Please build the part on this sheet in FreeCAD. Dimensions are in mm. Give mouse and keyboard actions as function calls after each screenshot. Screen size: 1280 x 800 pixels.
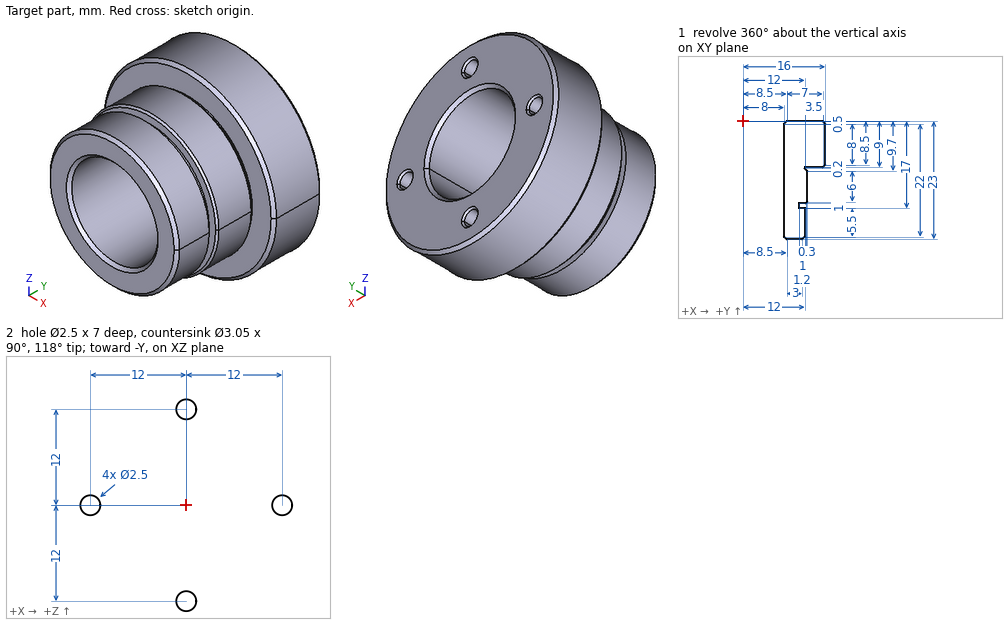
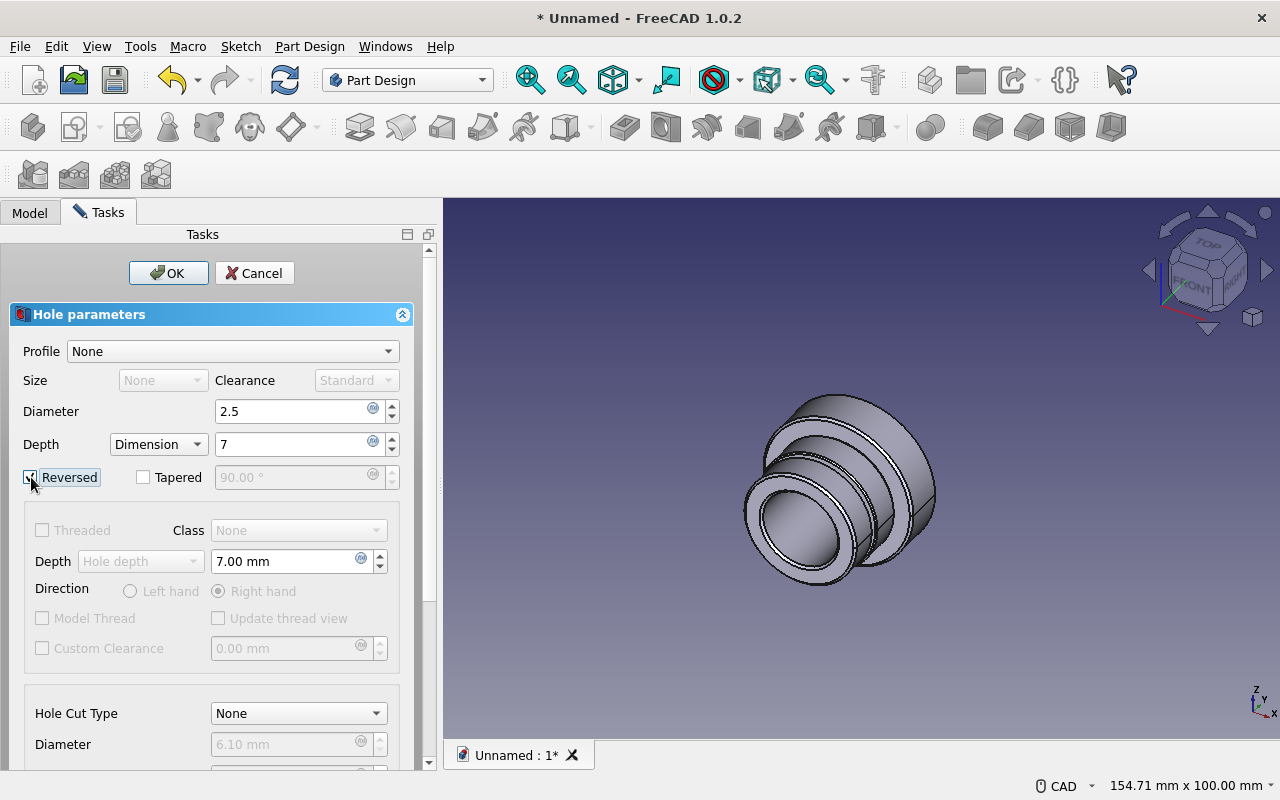
click(300, 714)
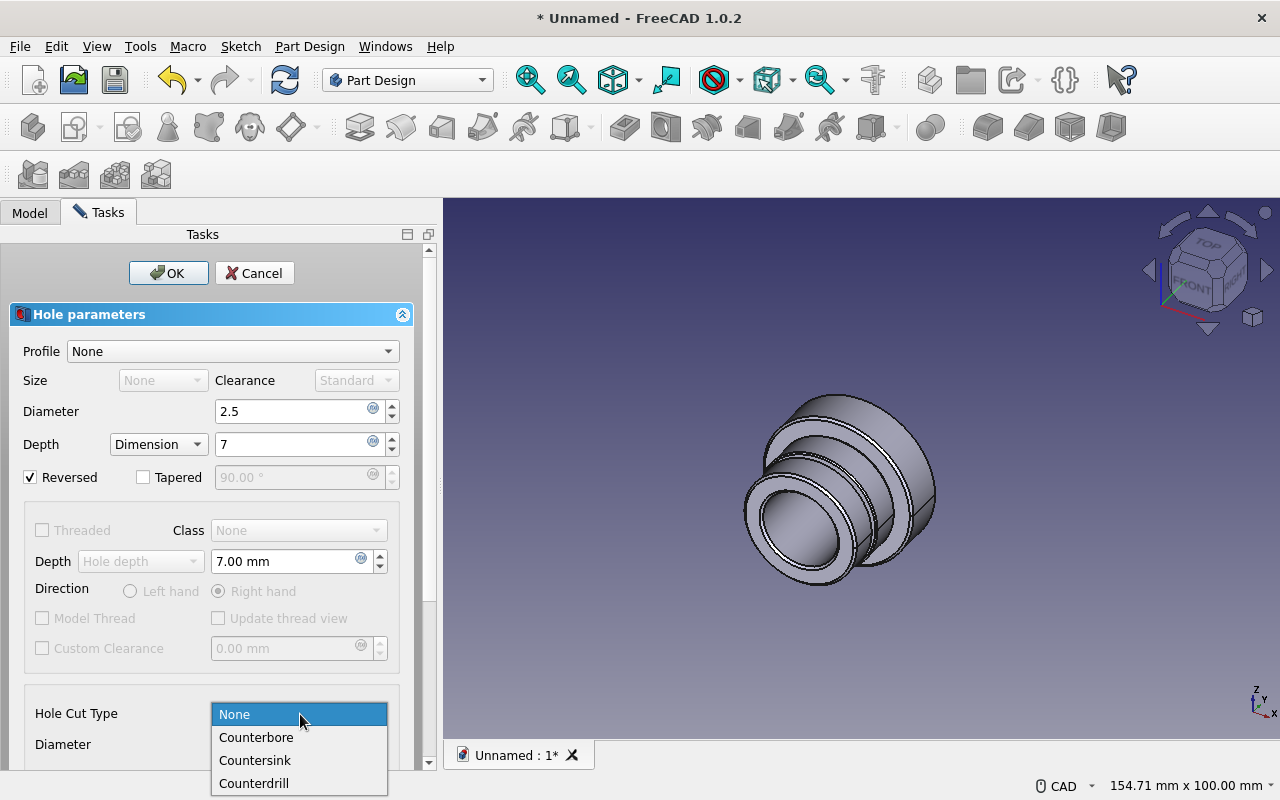
click(298, 760)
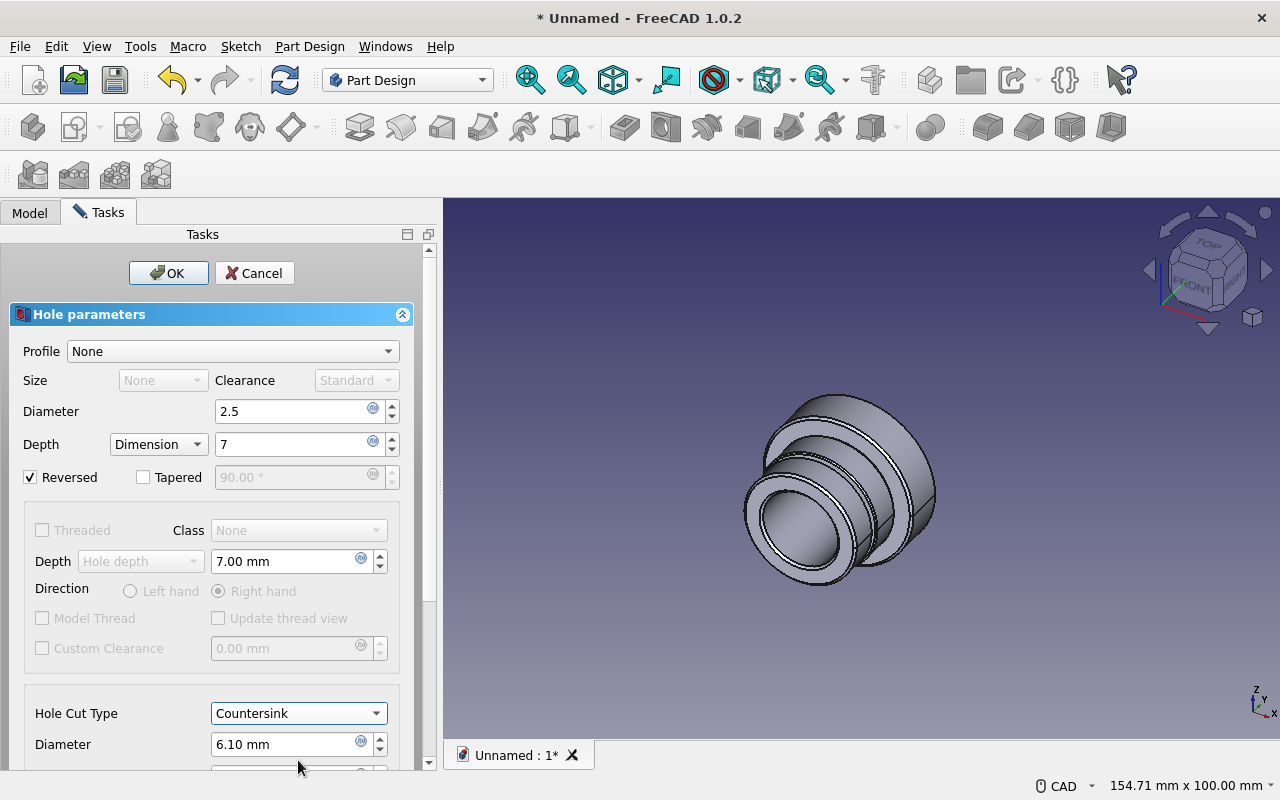
triple_click(292, 744)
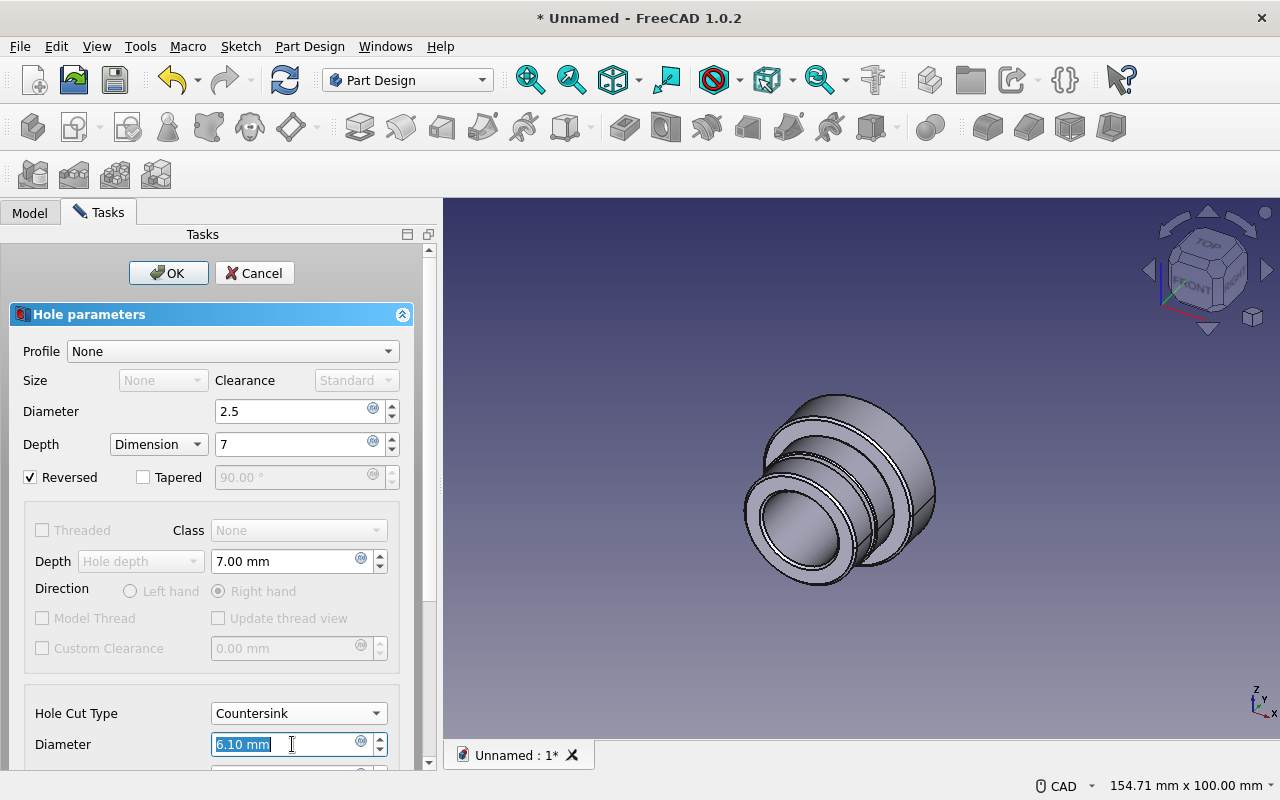
text(3.05)
key(Tab)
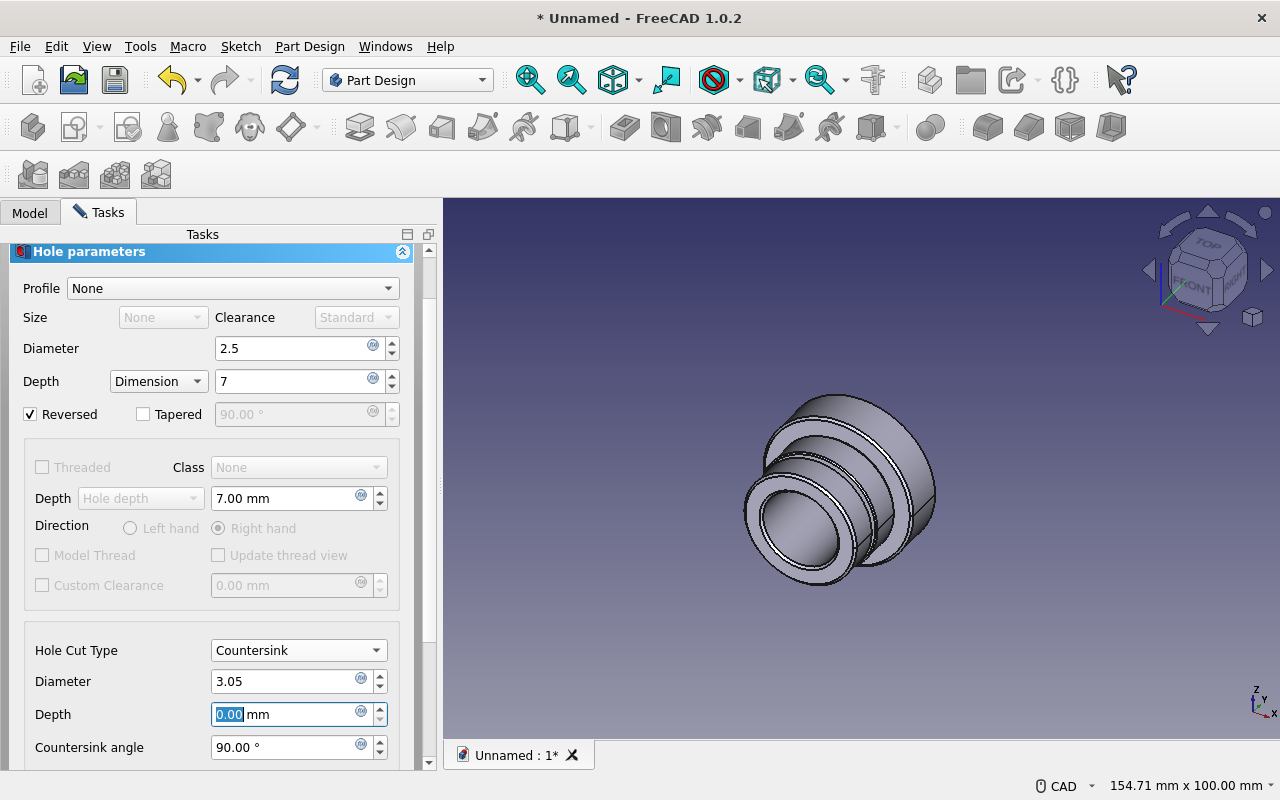
scroll(429, 507, up, 2)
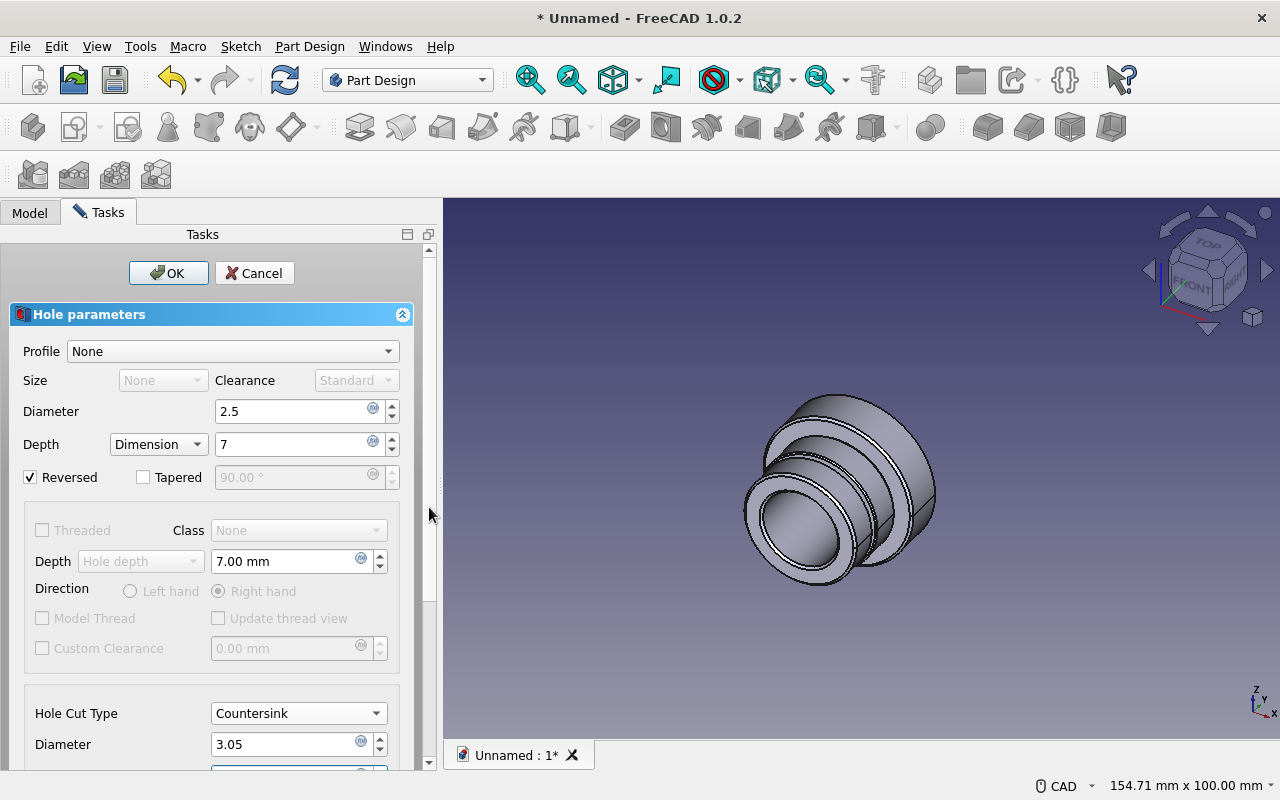
click(169, 273)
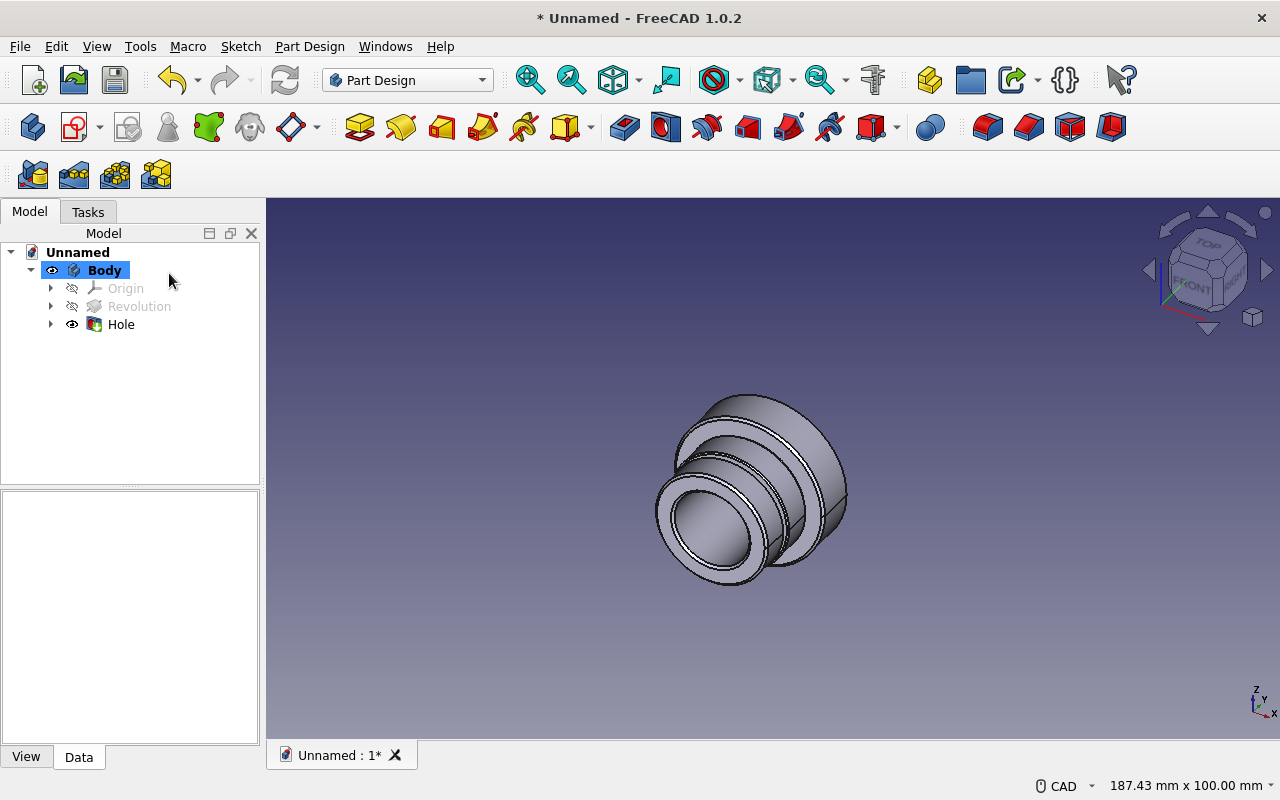
key(0)